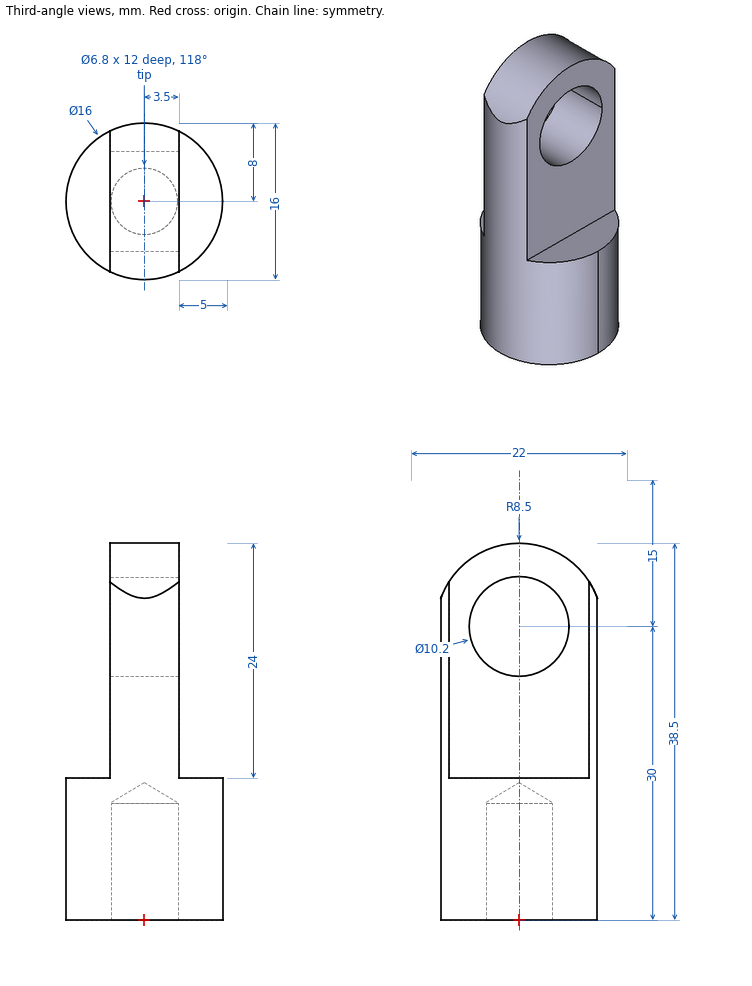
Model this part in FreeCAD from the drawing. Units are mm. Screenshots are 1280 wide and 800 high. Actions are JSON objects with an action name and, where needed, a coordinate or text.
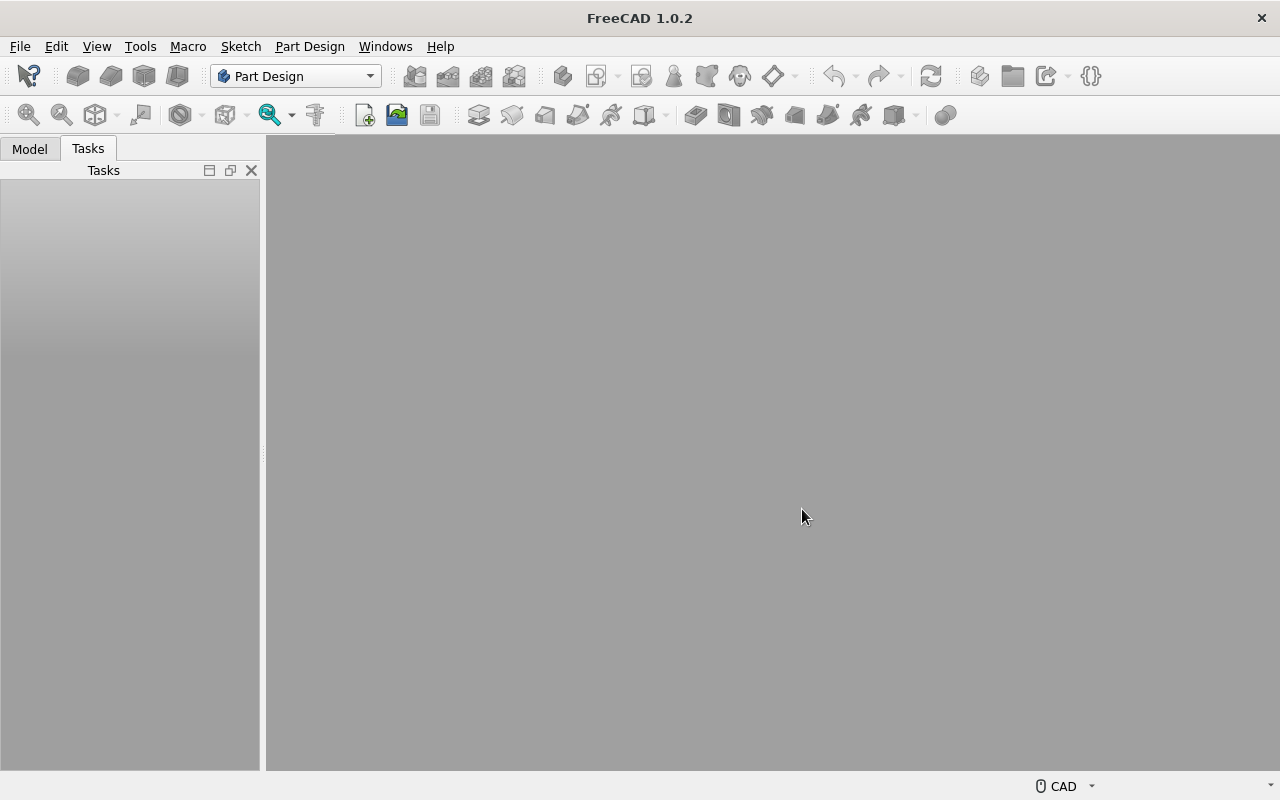
{"action": "left_click", "coordinate": [364, 116]}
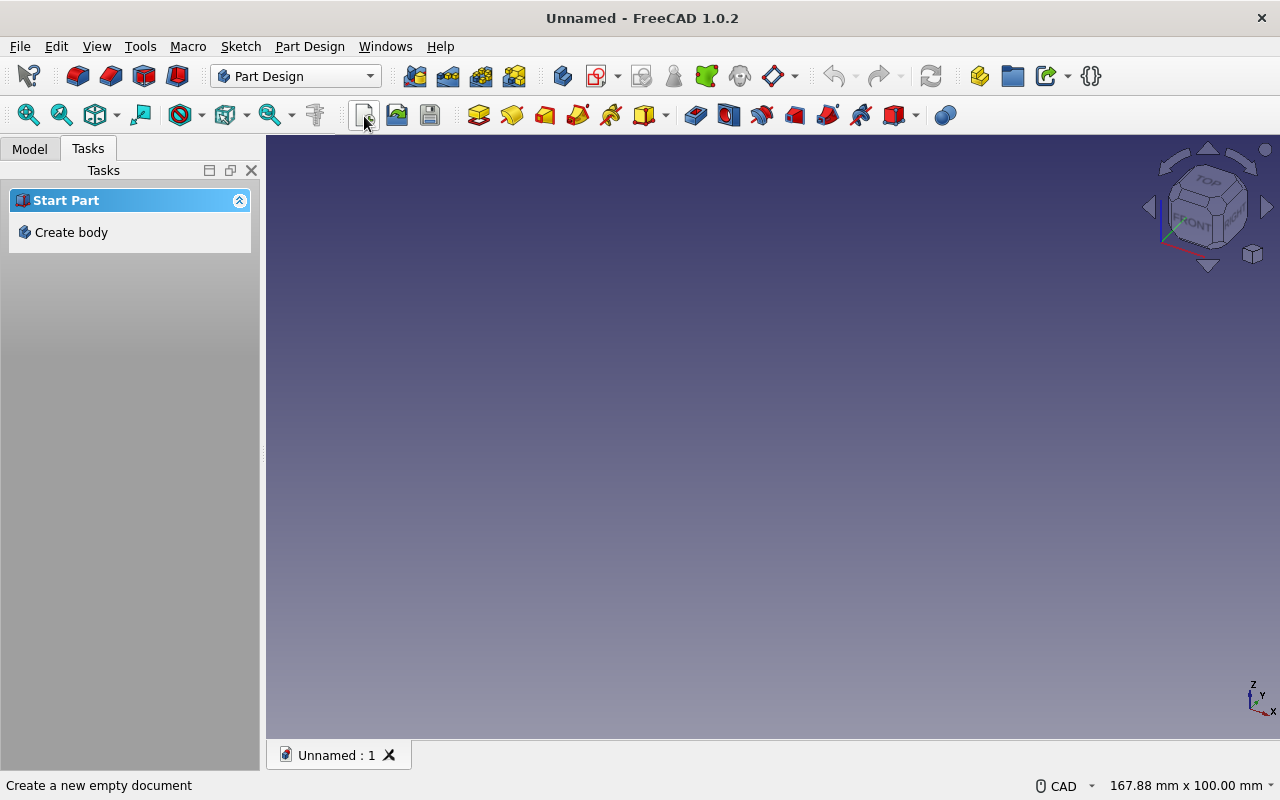
{"action": "left_click", "coordinate": [596, 76]}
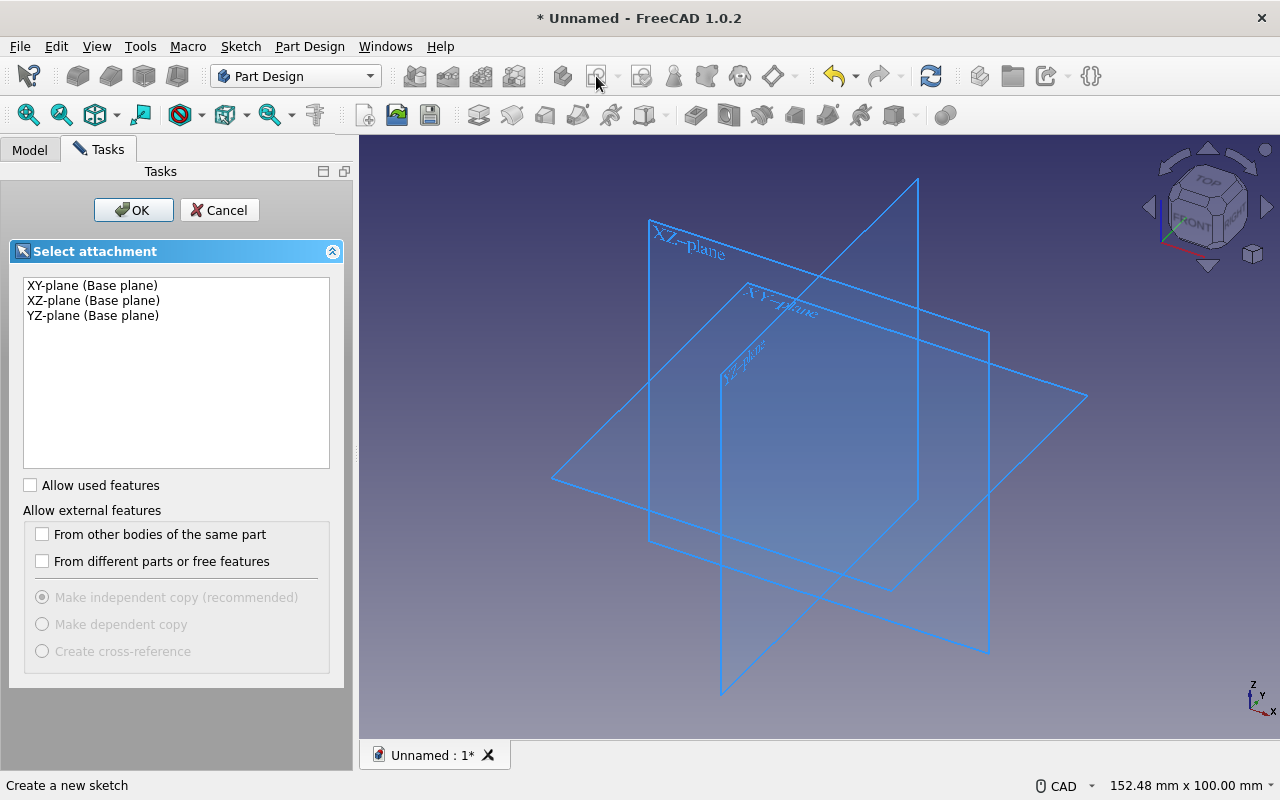
{"action": "left_click", "coordinate": [84, 286]}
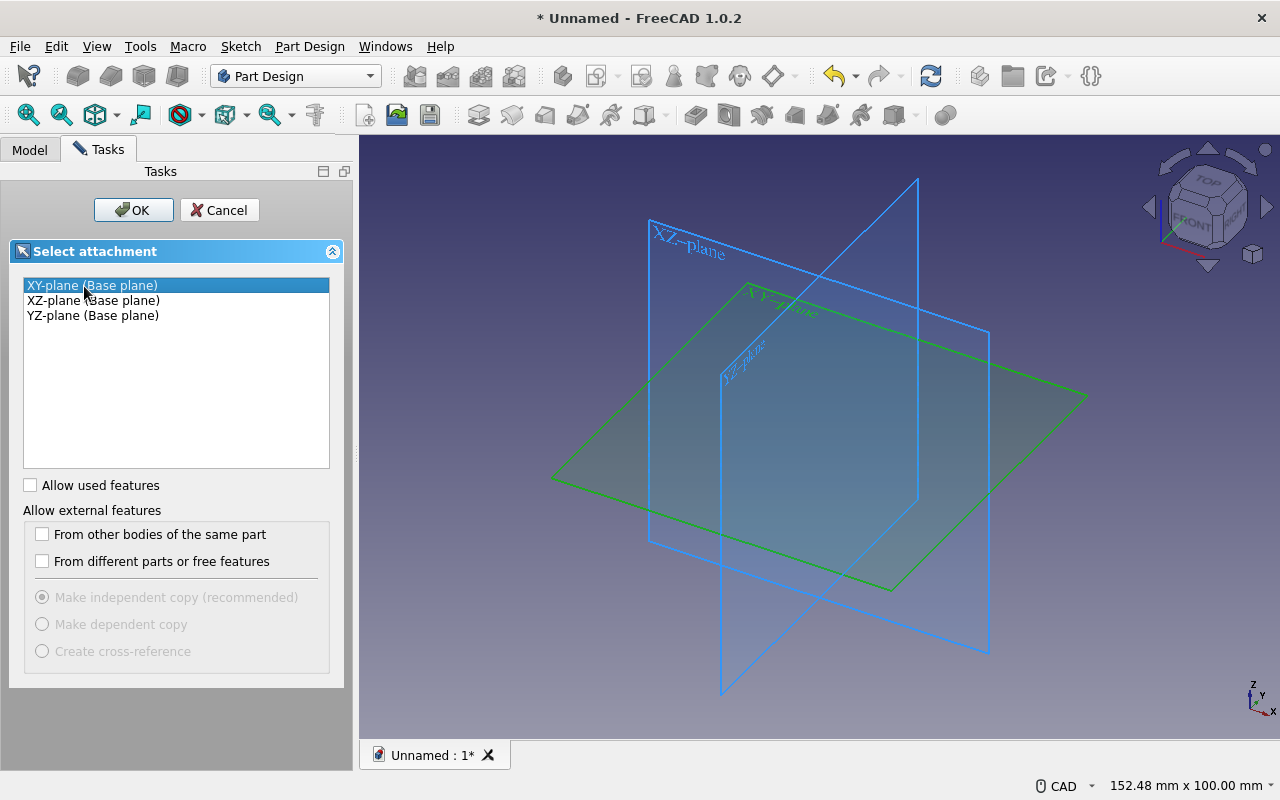
{"action": "left_click", "coordinate": [134, 210]}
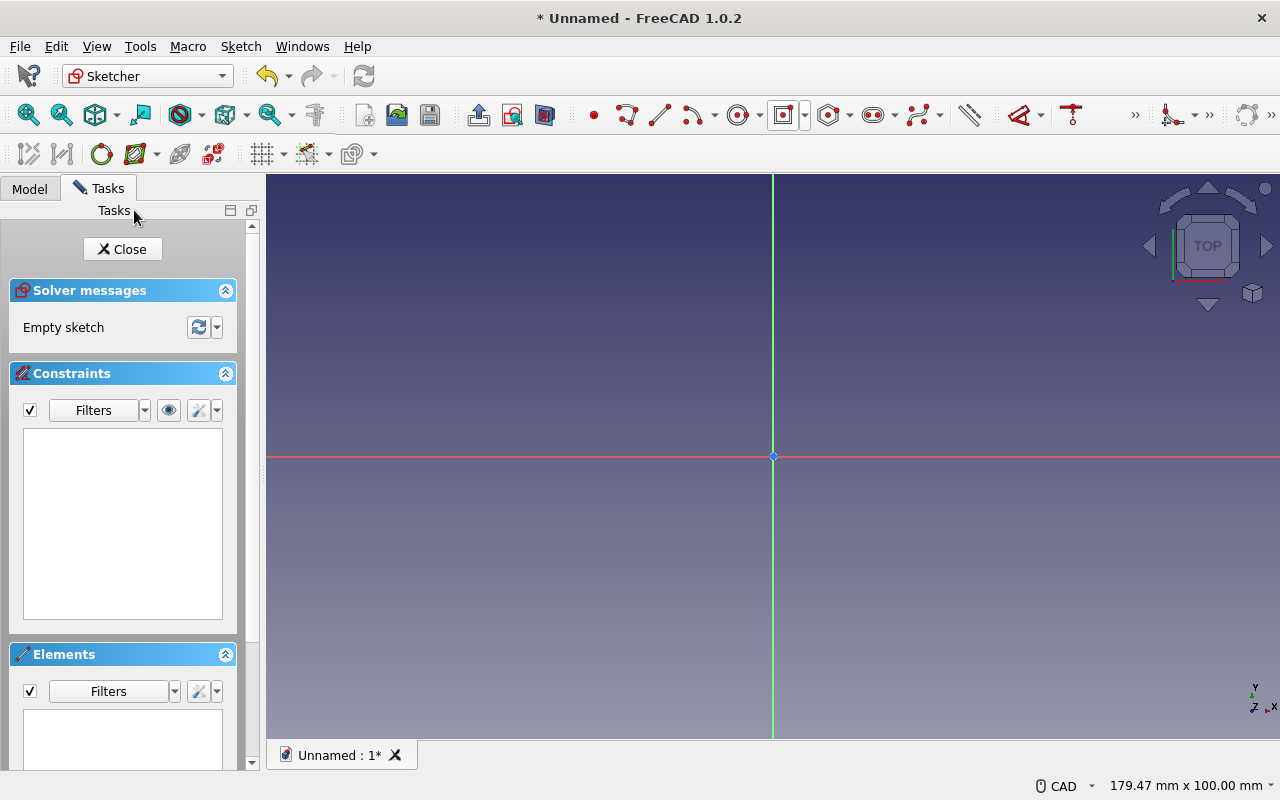
{"action": "scroll", "coordinate": [795, 456], "scroll_direction": "up", "scroll_amount": 7}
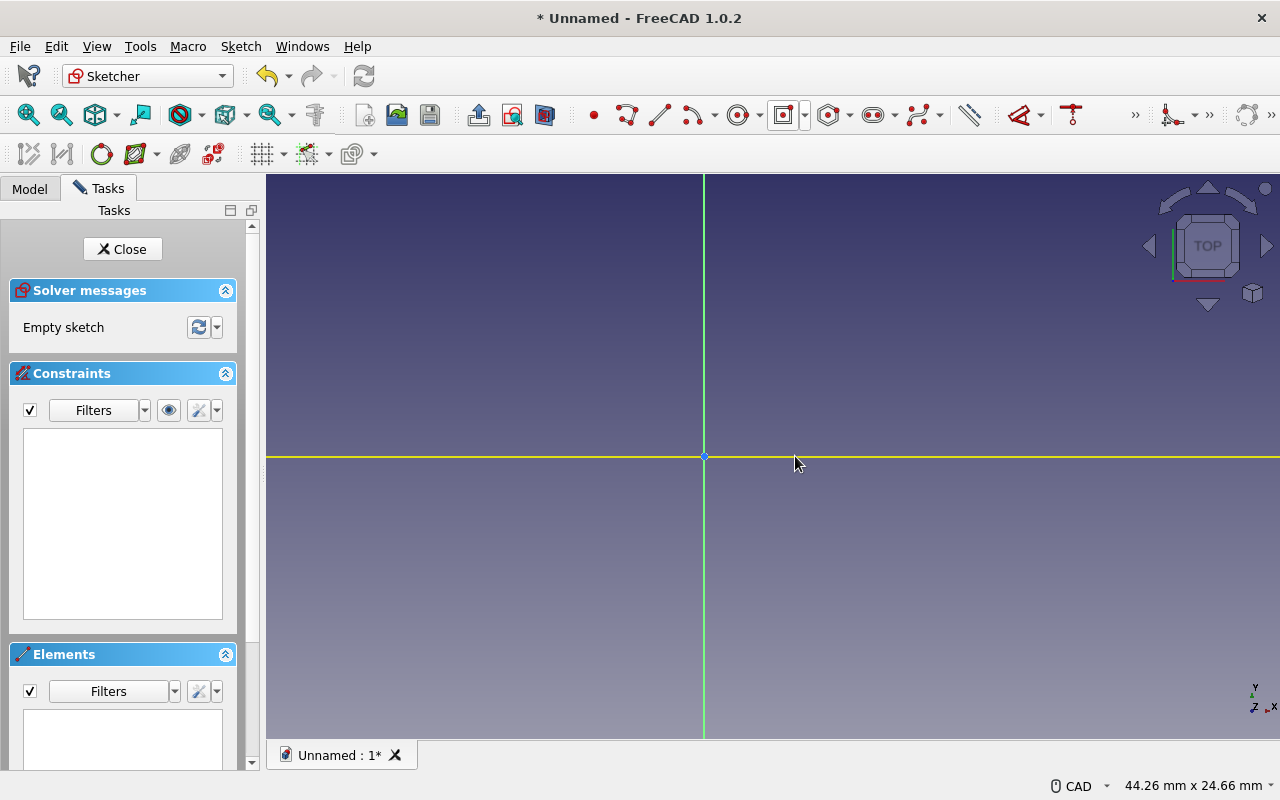
{"action": "key", "text": "g c"}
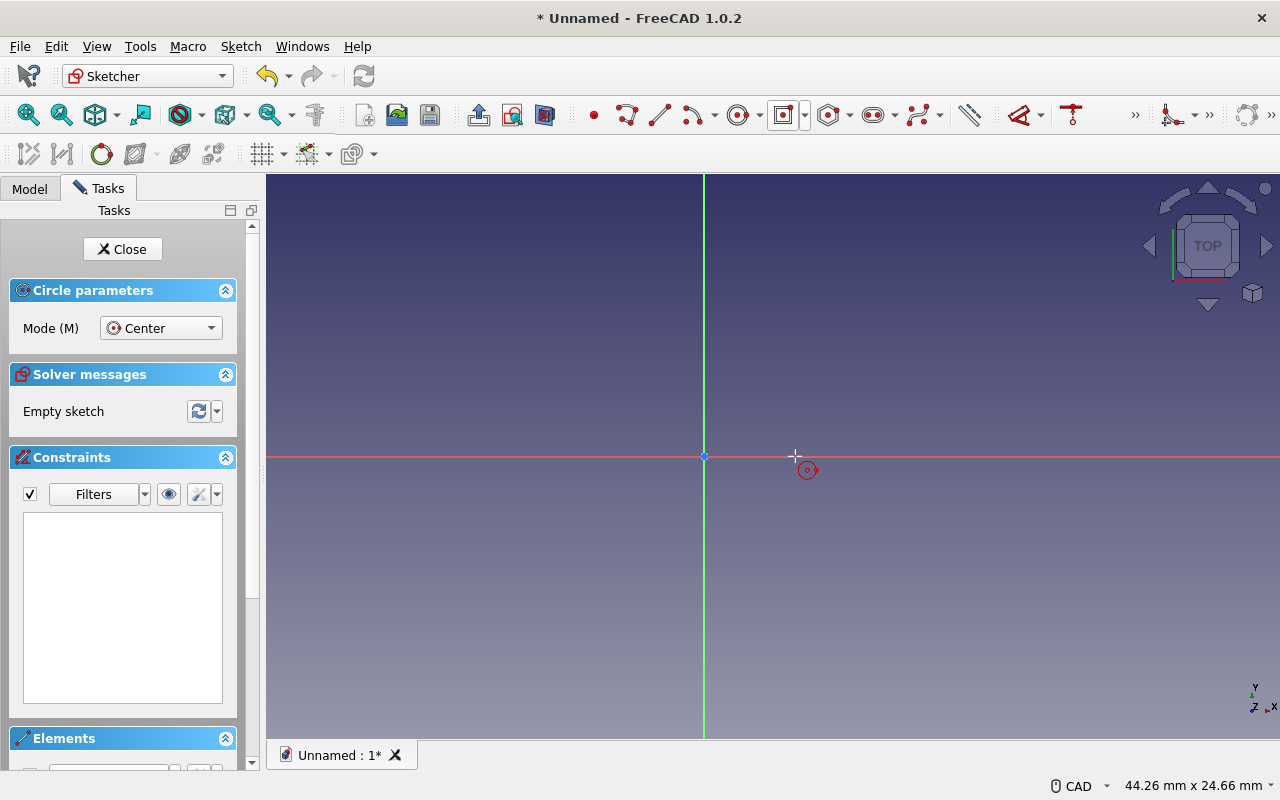
{"action": "left_click", "coordinate": [704, 456]}
{"action": "left_click", "coordinate": [834, 327]}
{"action": "key", "text": "Escape"}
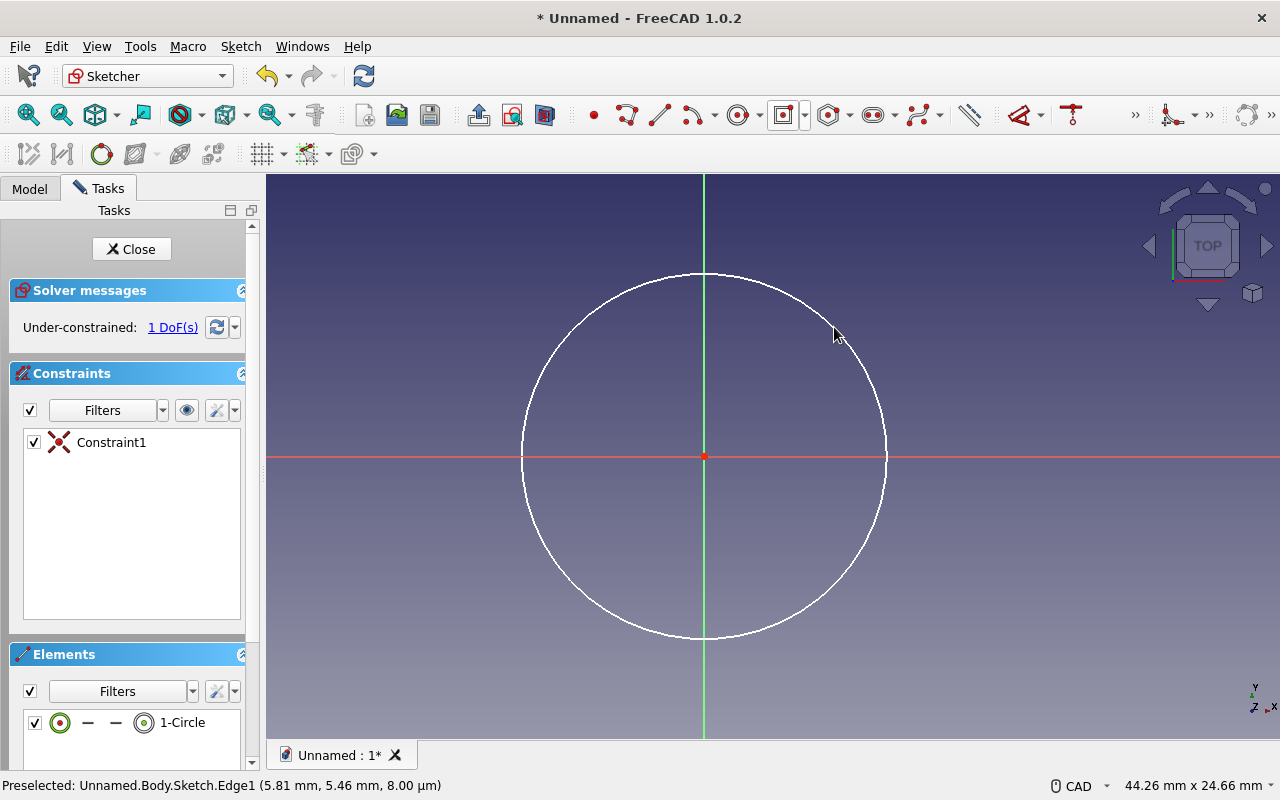
{"action": "key", "text": "d"}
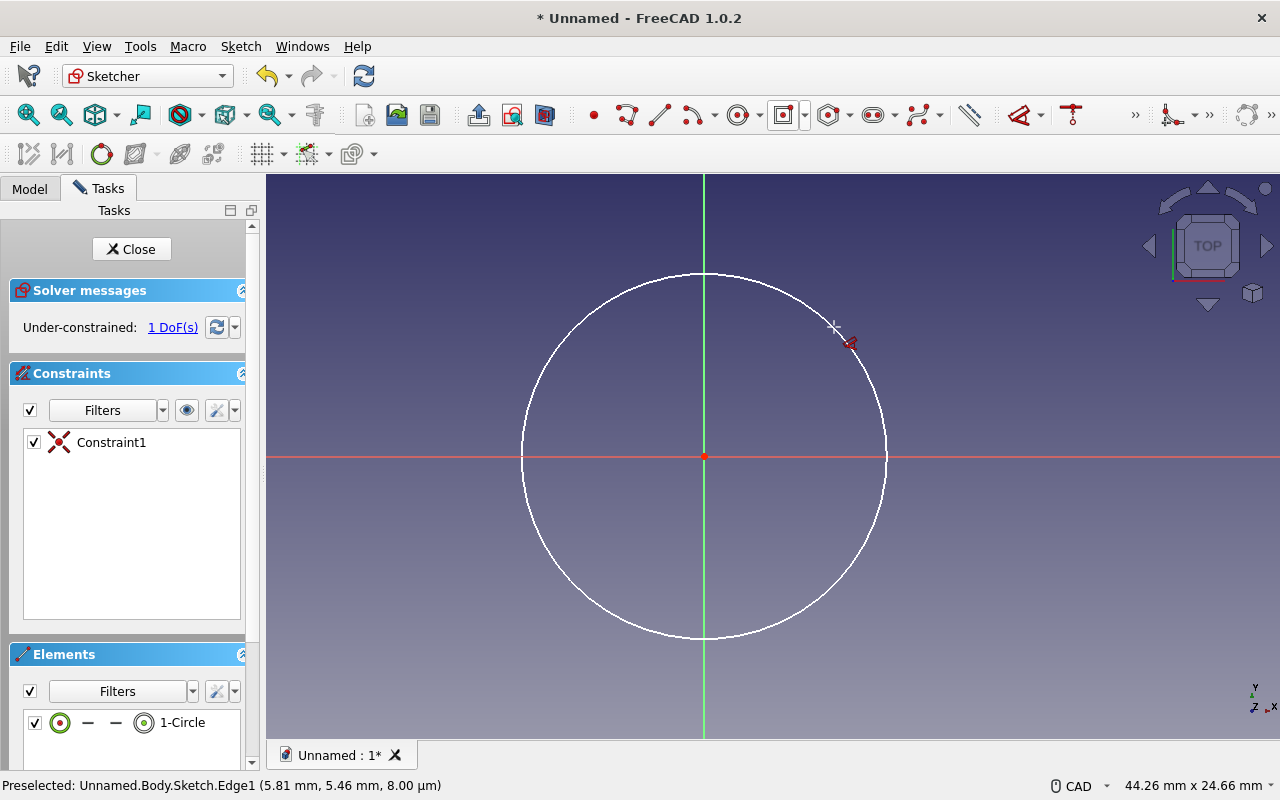
{"action": "left_click", "coordinate": [833, 327]}
{"action": "left_click", "coordinate": [856, 304]}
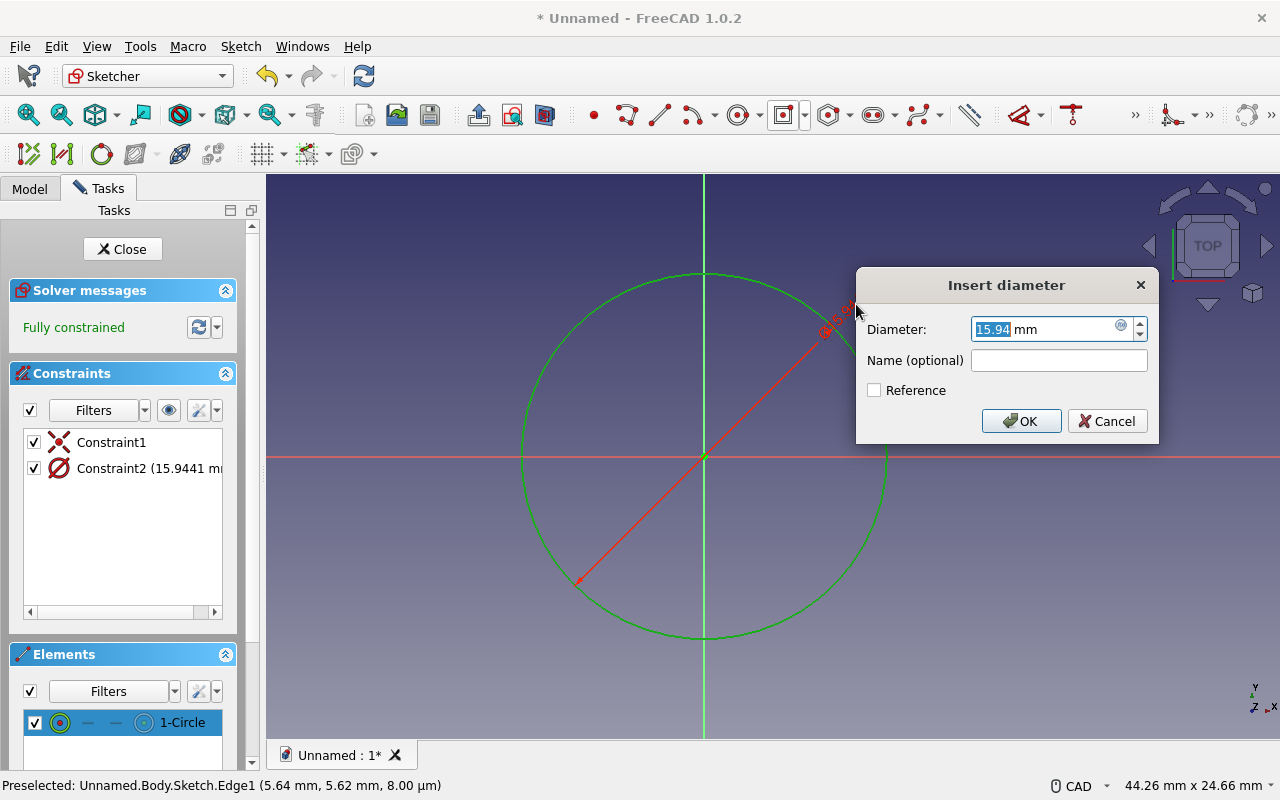
{"action": "type", "text": "16"}
{"action": "key", "text": "Return"}
{"action": "key", "text": "Escape"}